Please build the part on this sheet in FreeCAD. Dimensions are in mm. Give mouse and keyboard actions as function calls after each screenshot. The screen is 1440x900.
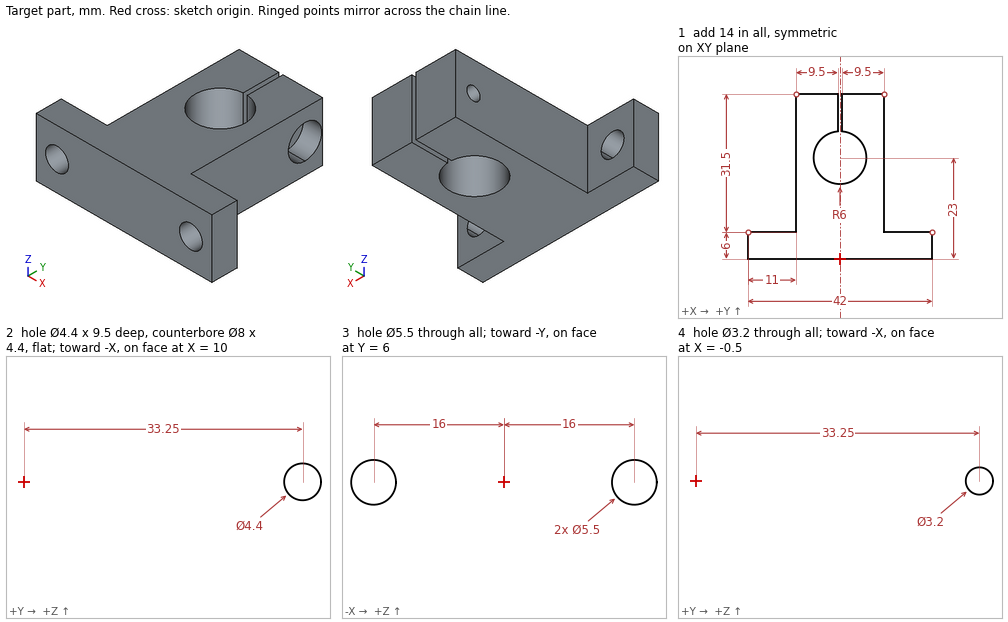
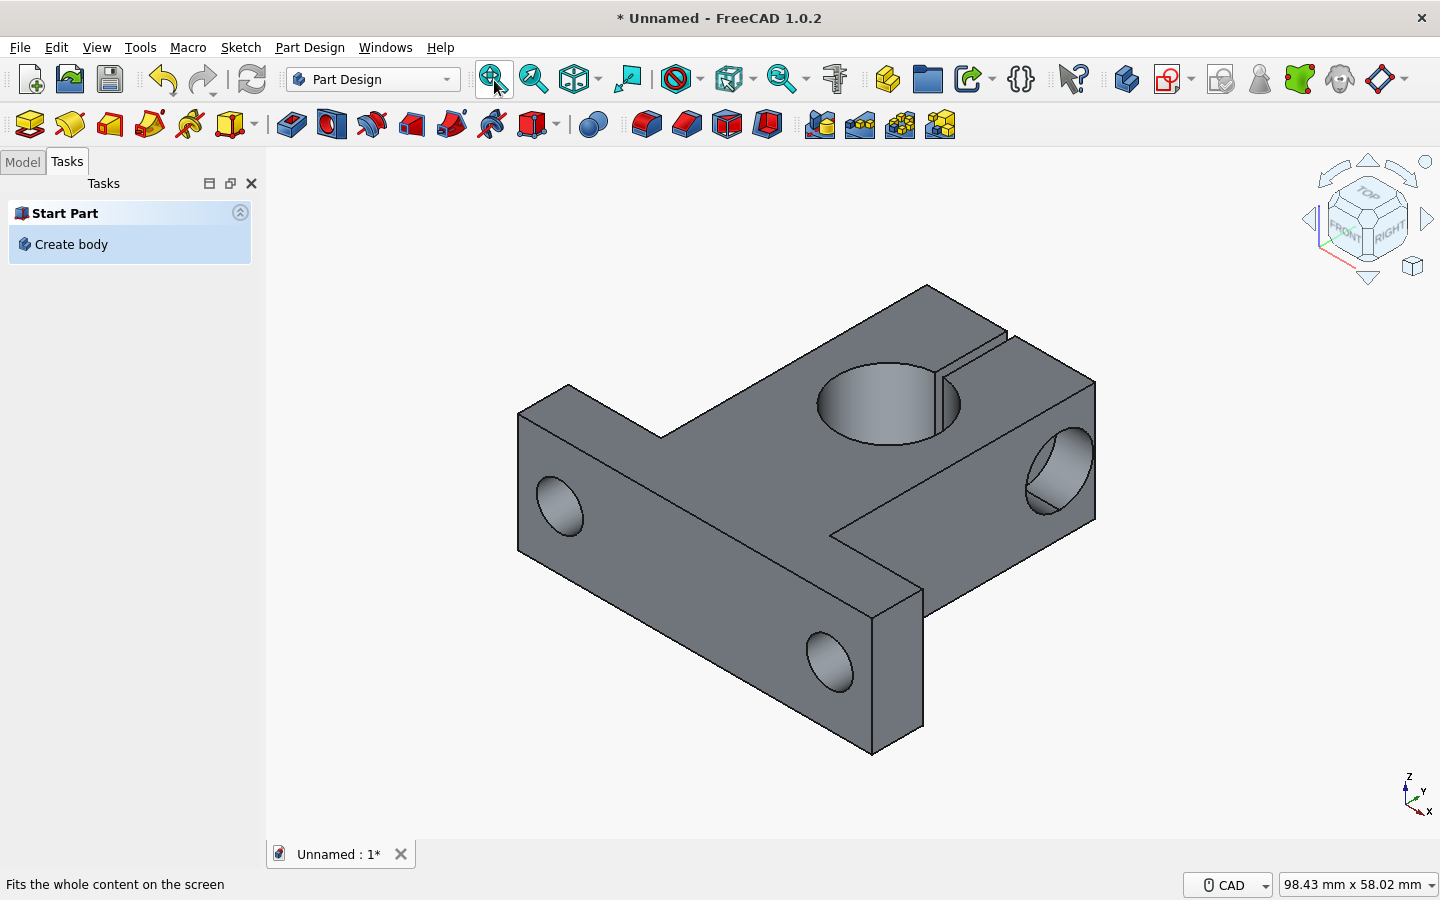
key(3)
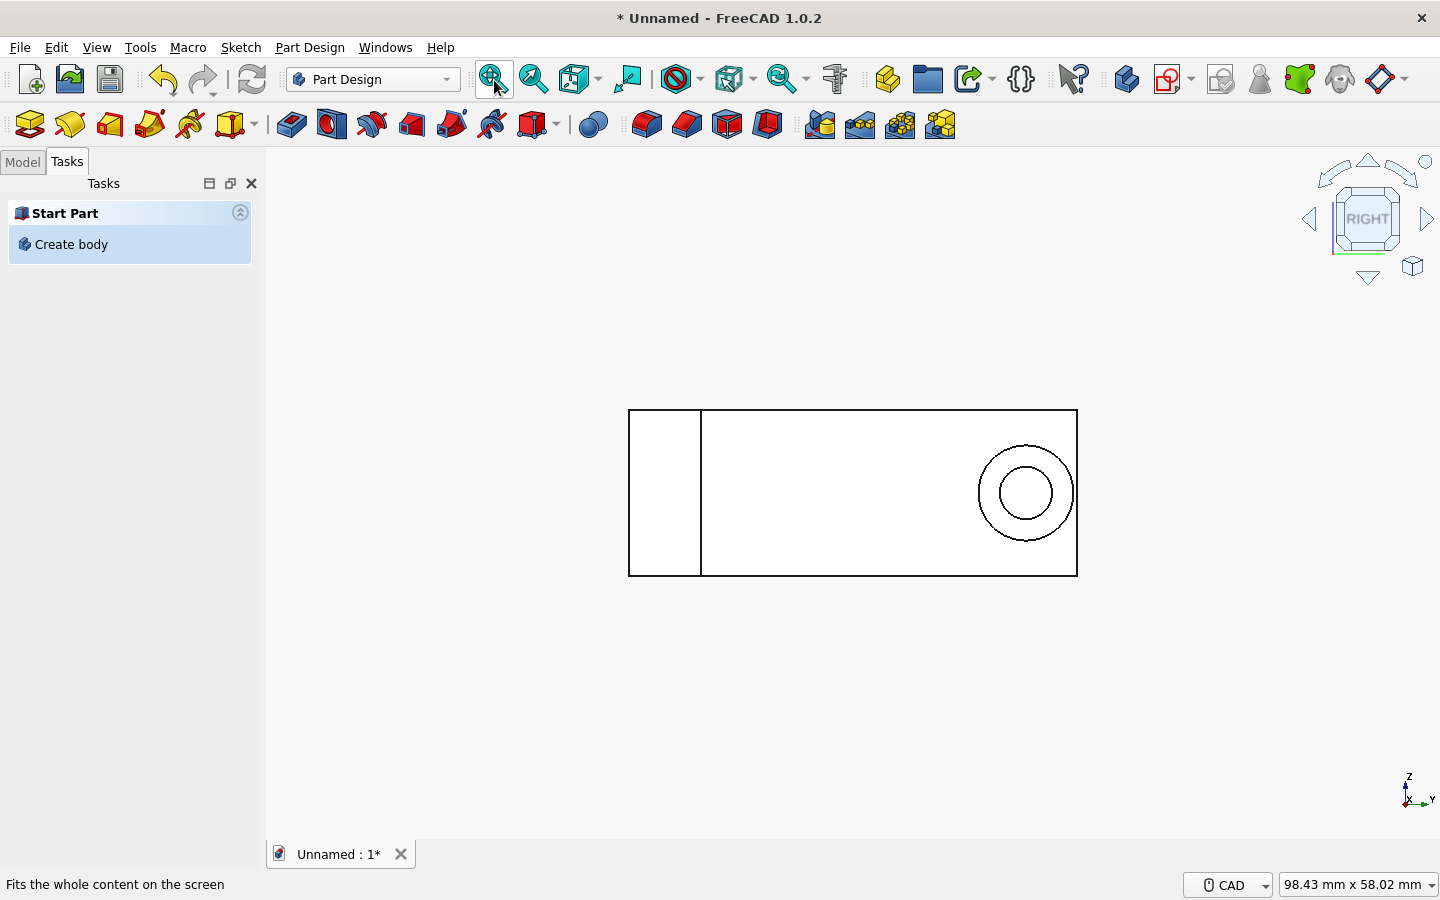
click(494, 80)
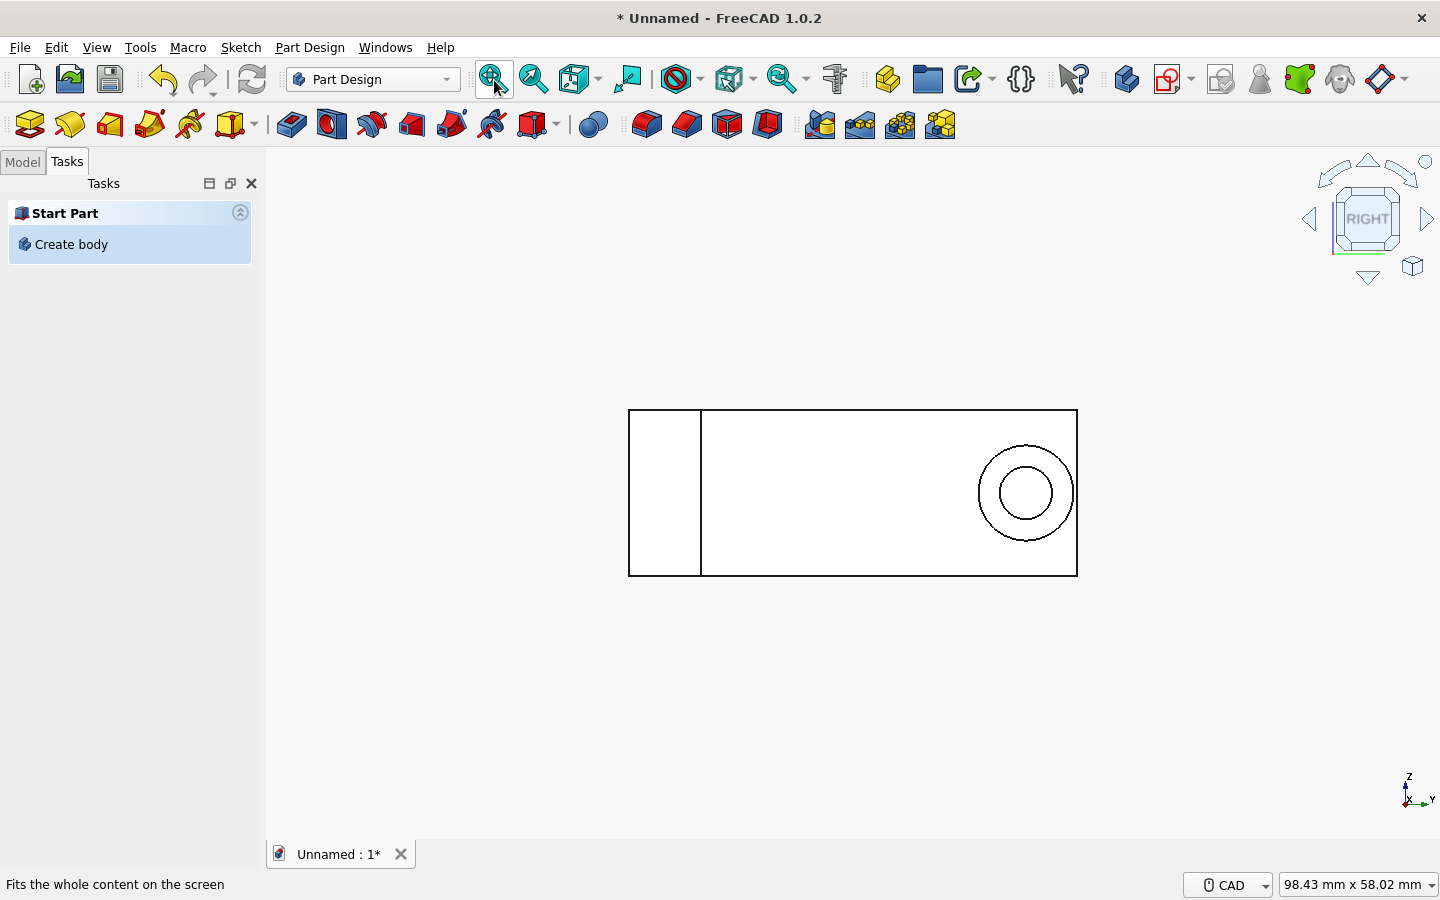
click(1026, 492)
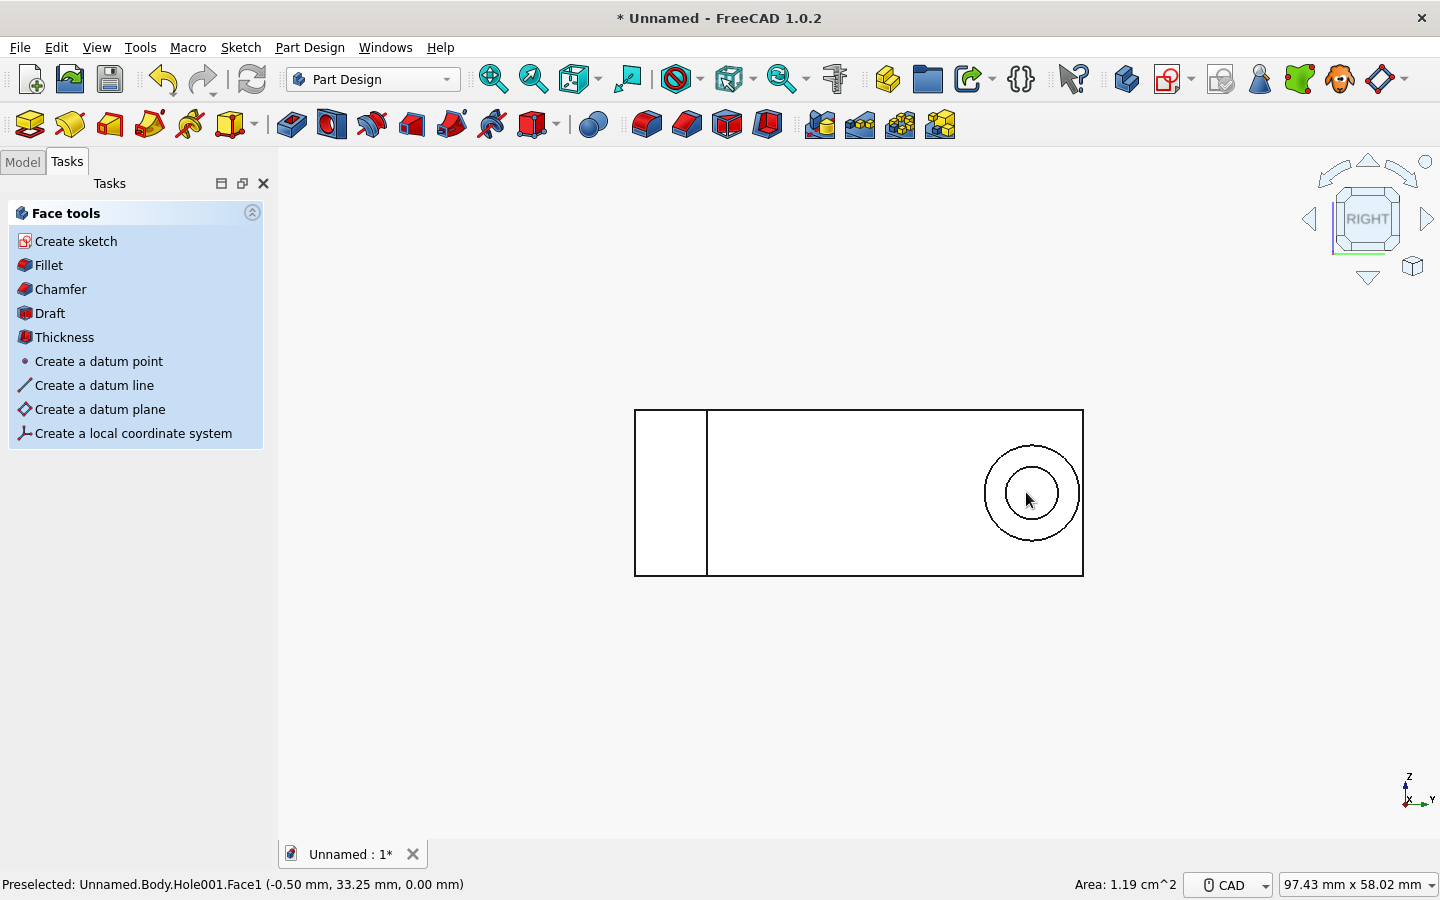
click(1168, 80)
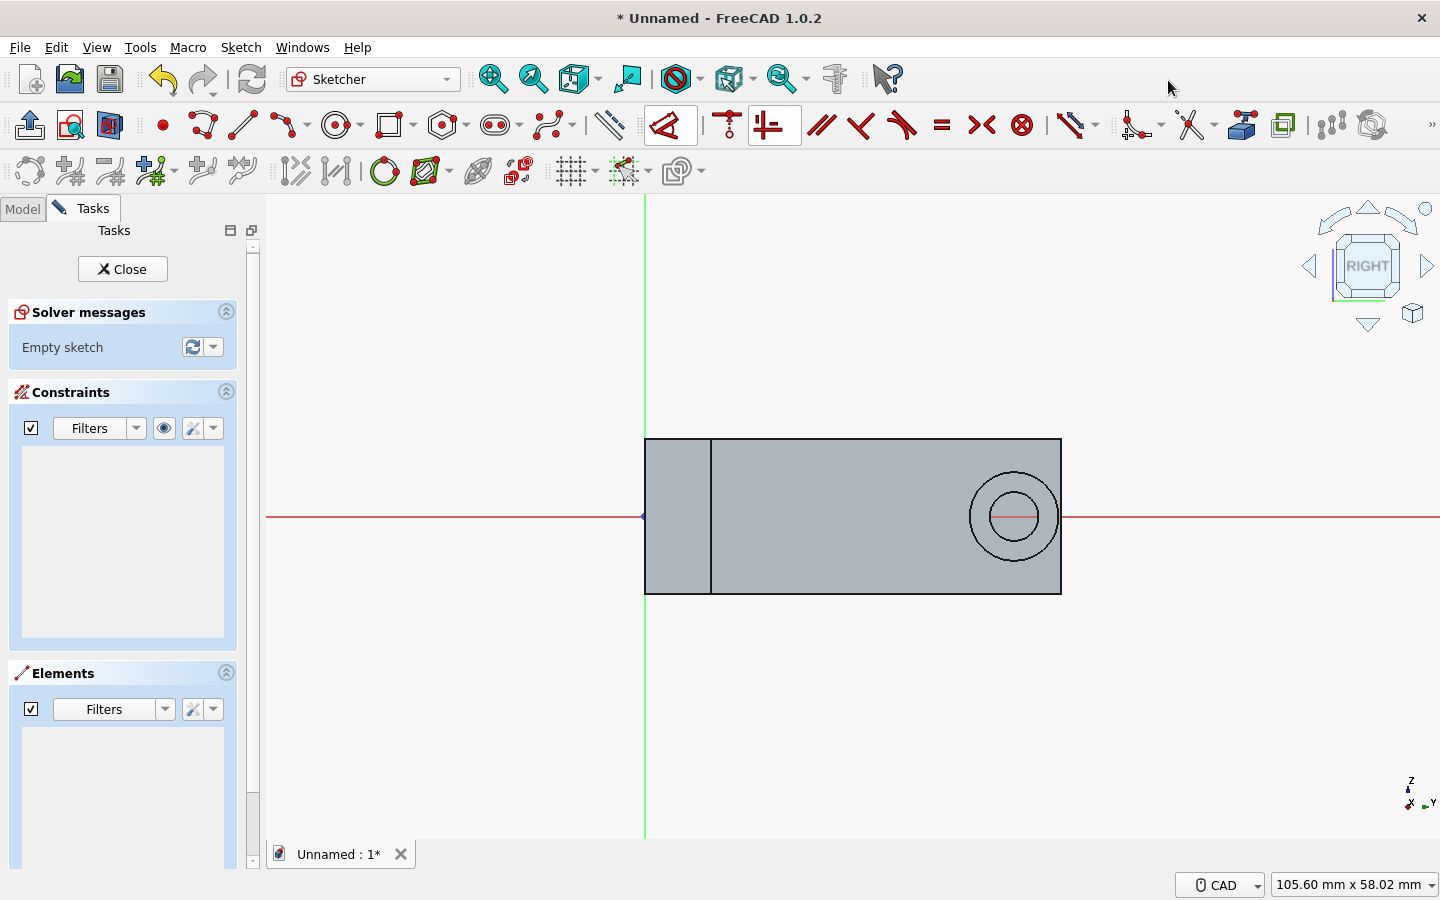
scroll(1037, 516, up, 12)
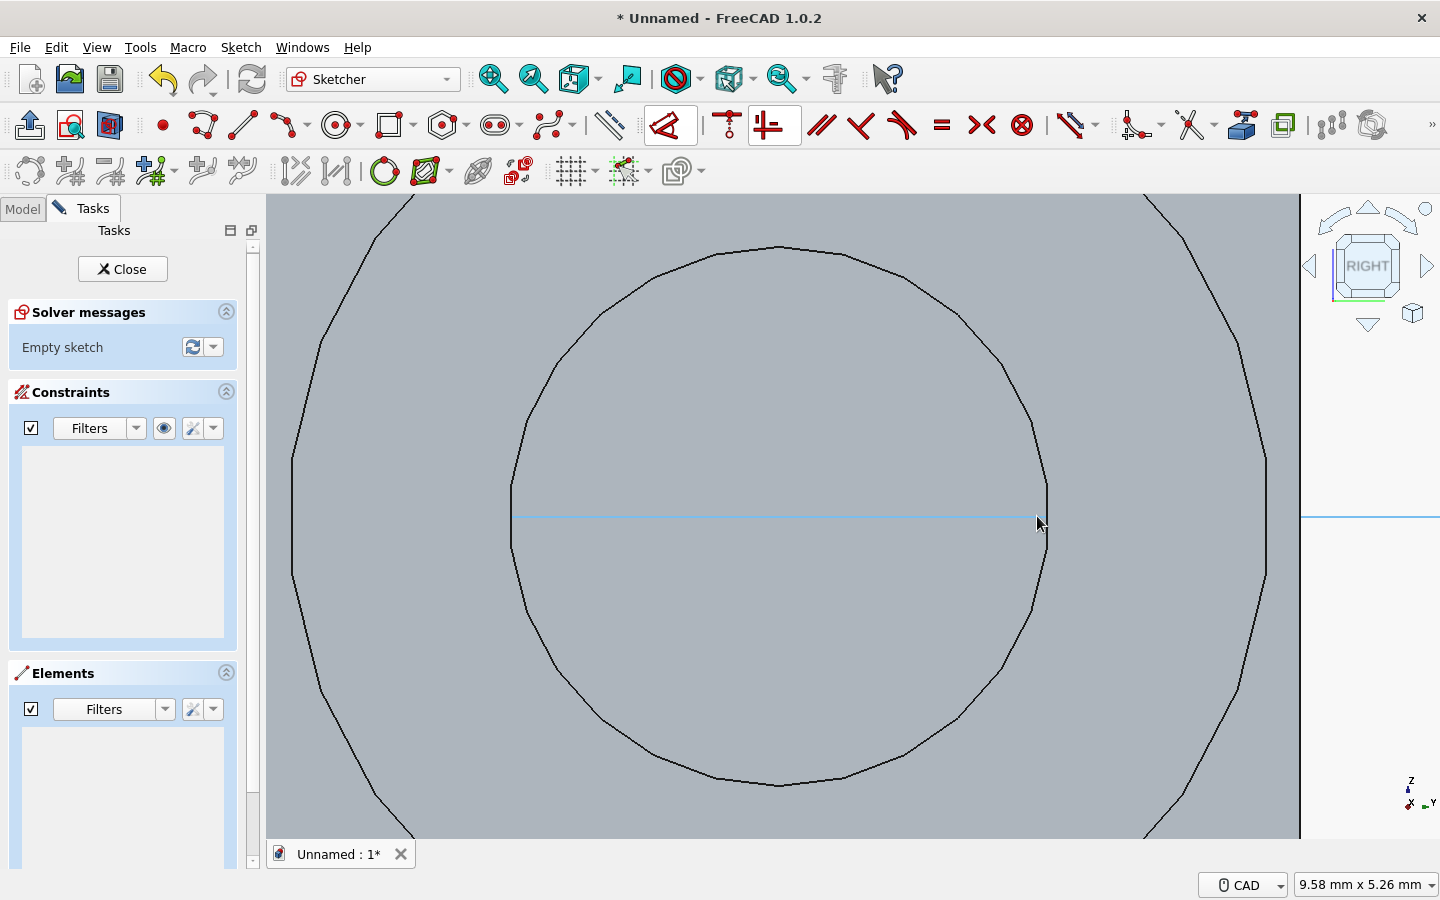
click(336, 126)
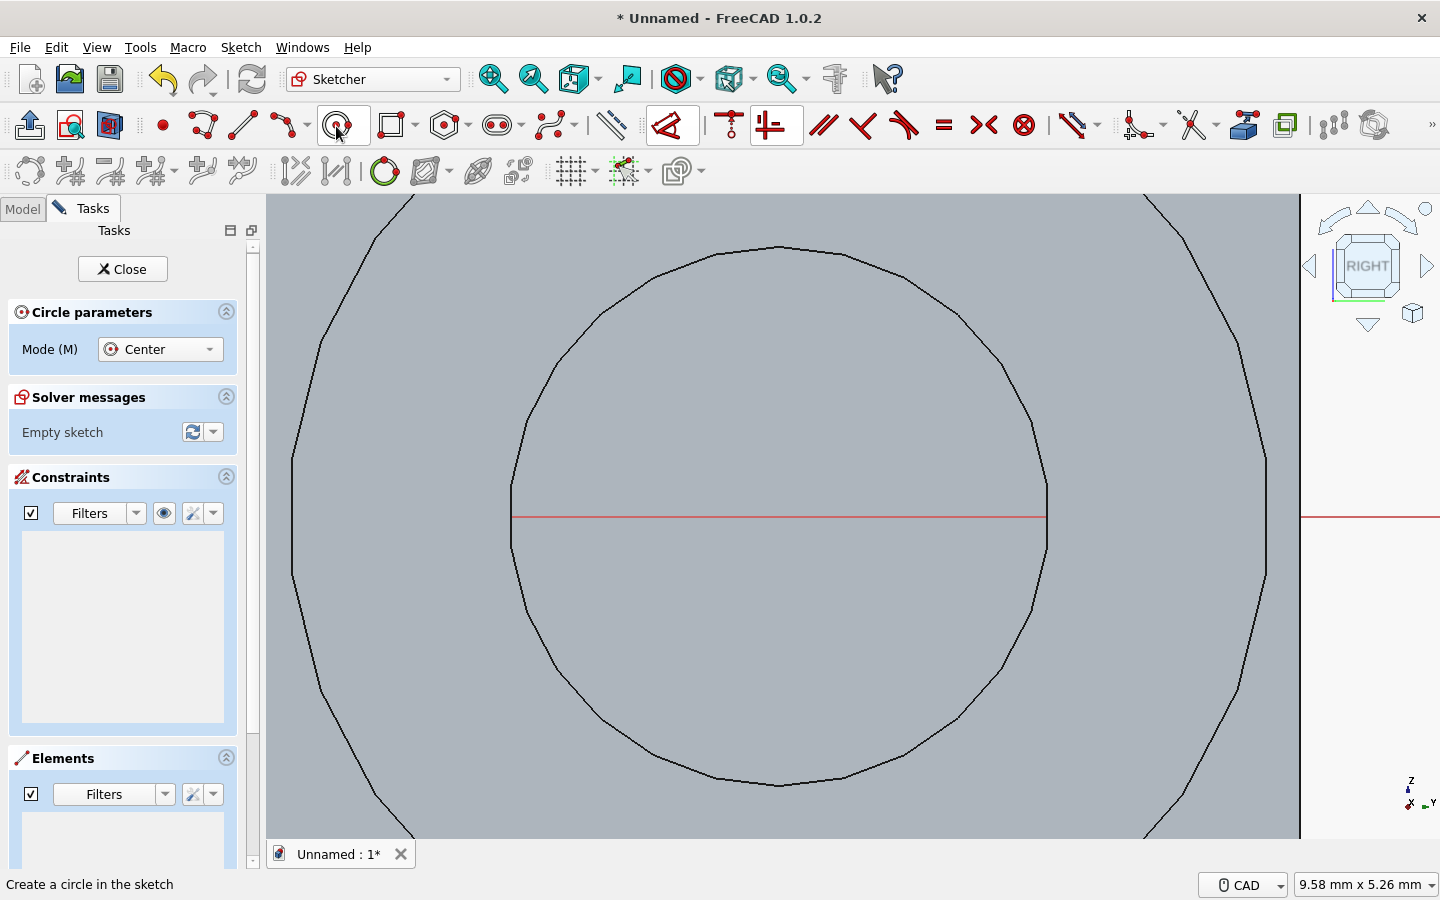
click(779, 516)
click(918, 378)
key(Escape)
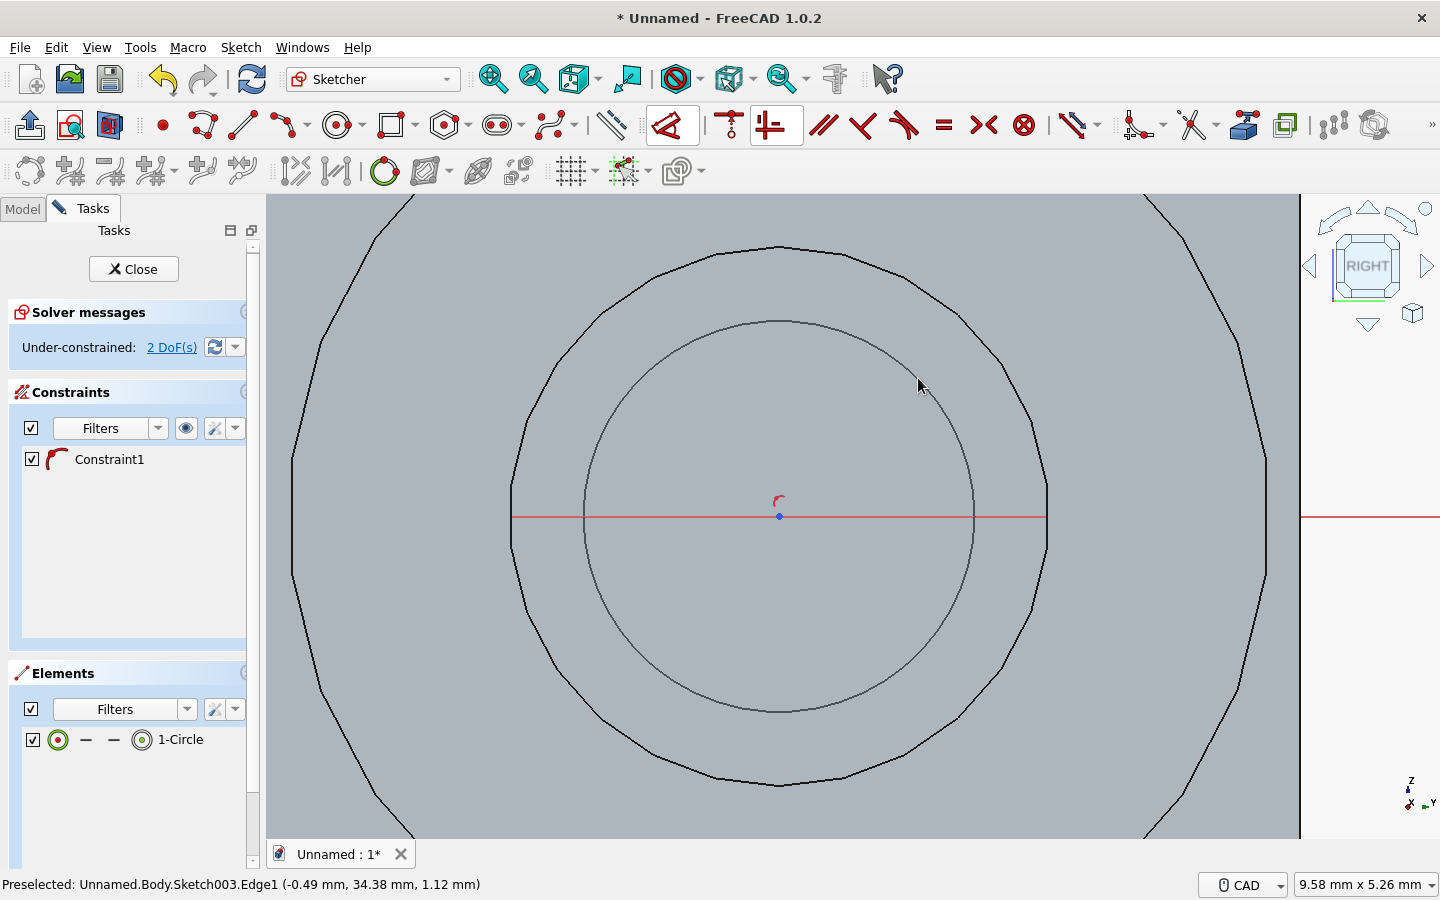
click(917, 378)